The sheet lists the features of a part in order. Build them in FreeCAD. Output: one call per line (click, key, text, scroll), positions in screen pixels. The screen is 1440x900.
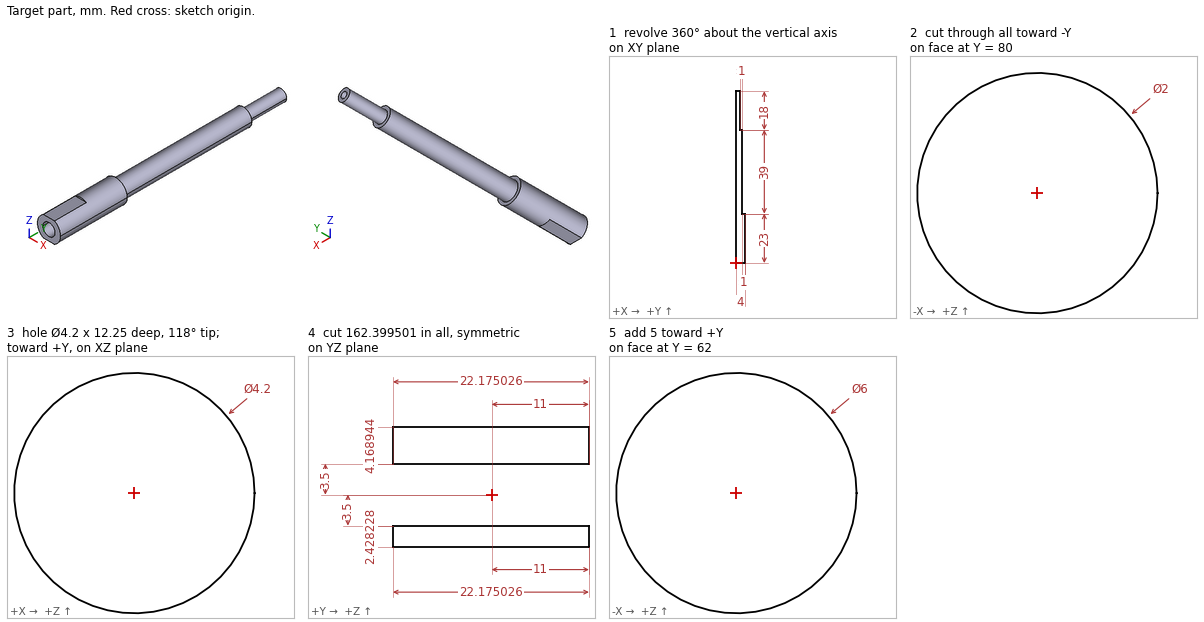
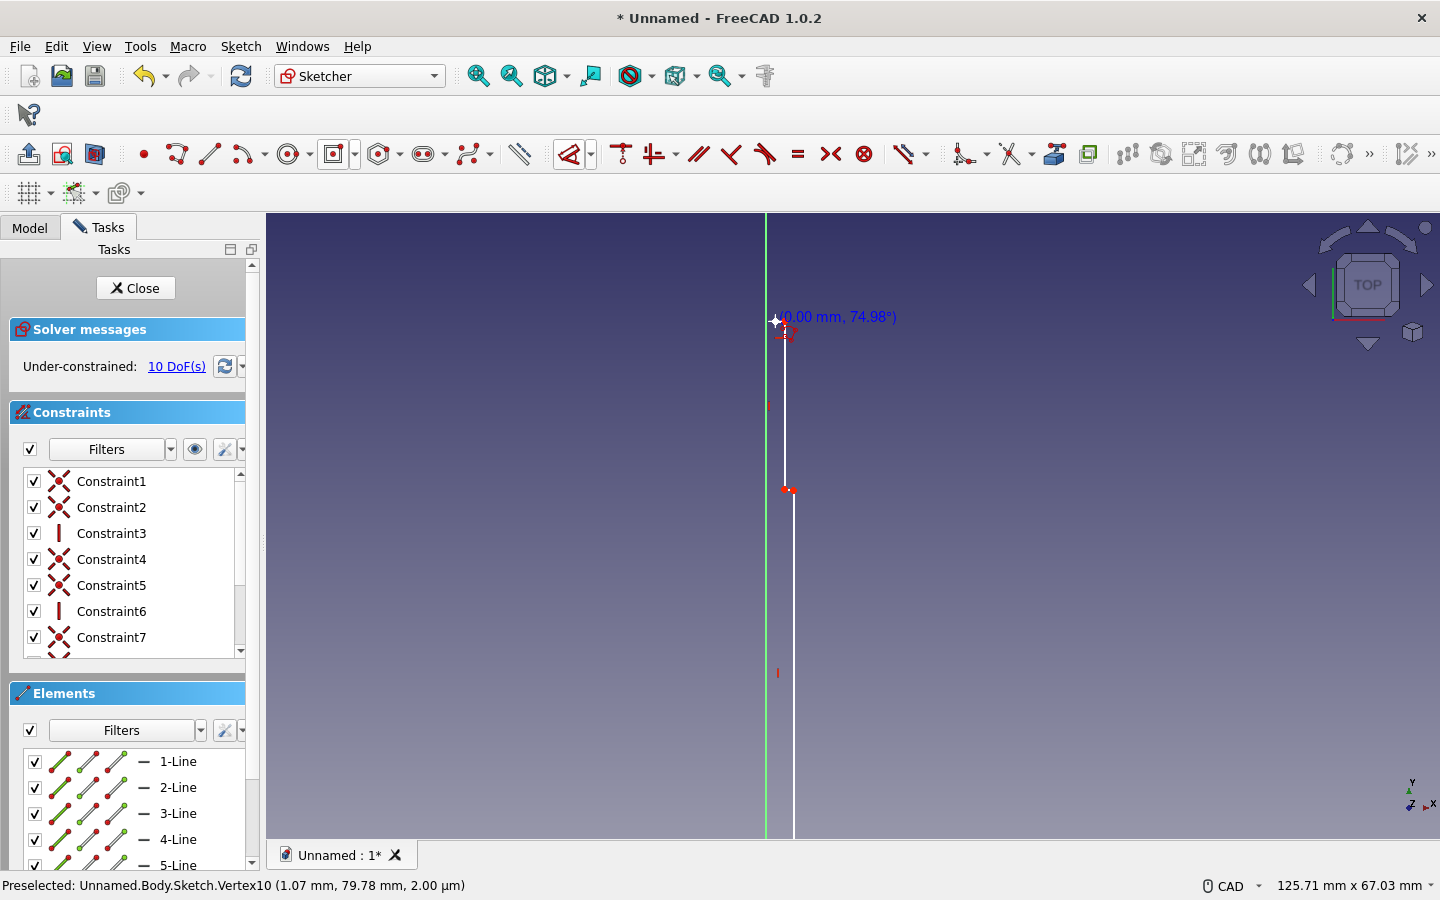
scroll(784, 321, down, 3)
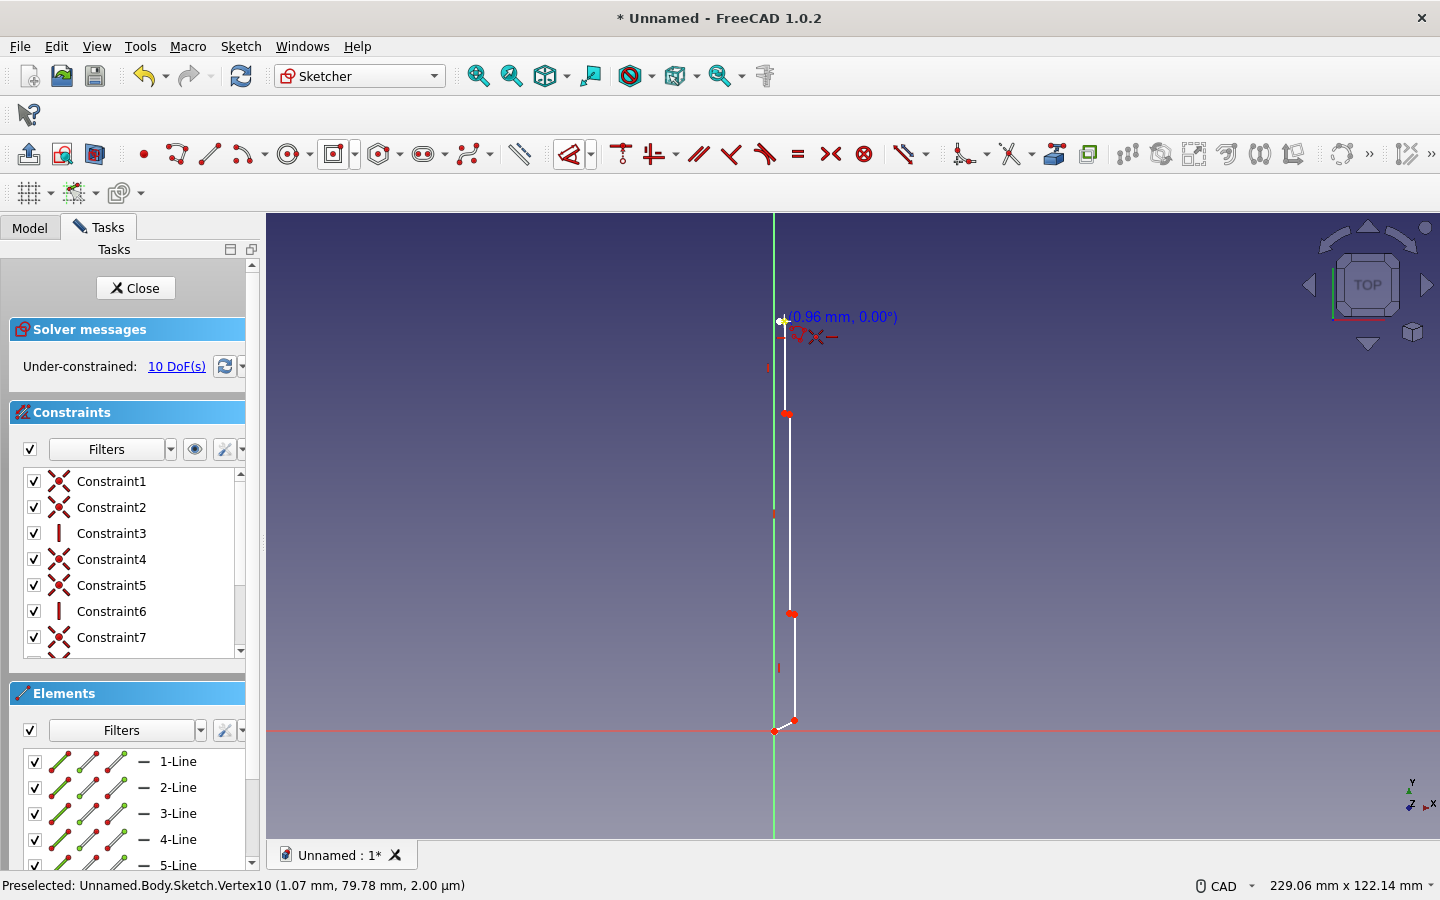
scroll(774, 731, up, 3)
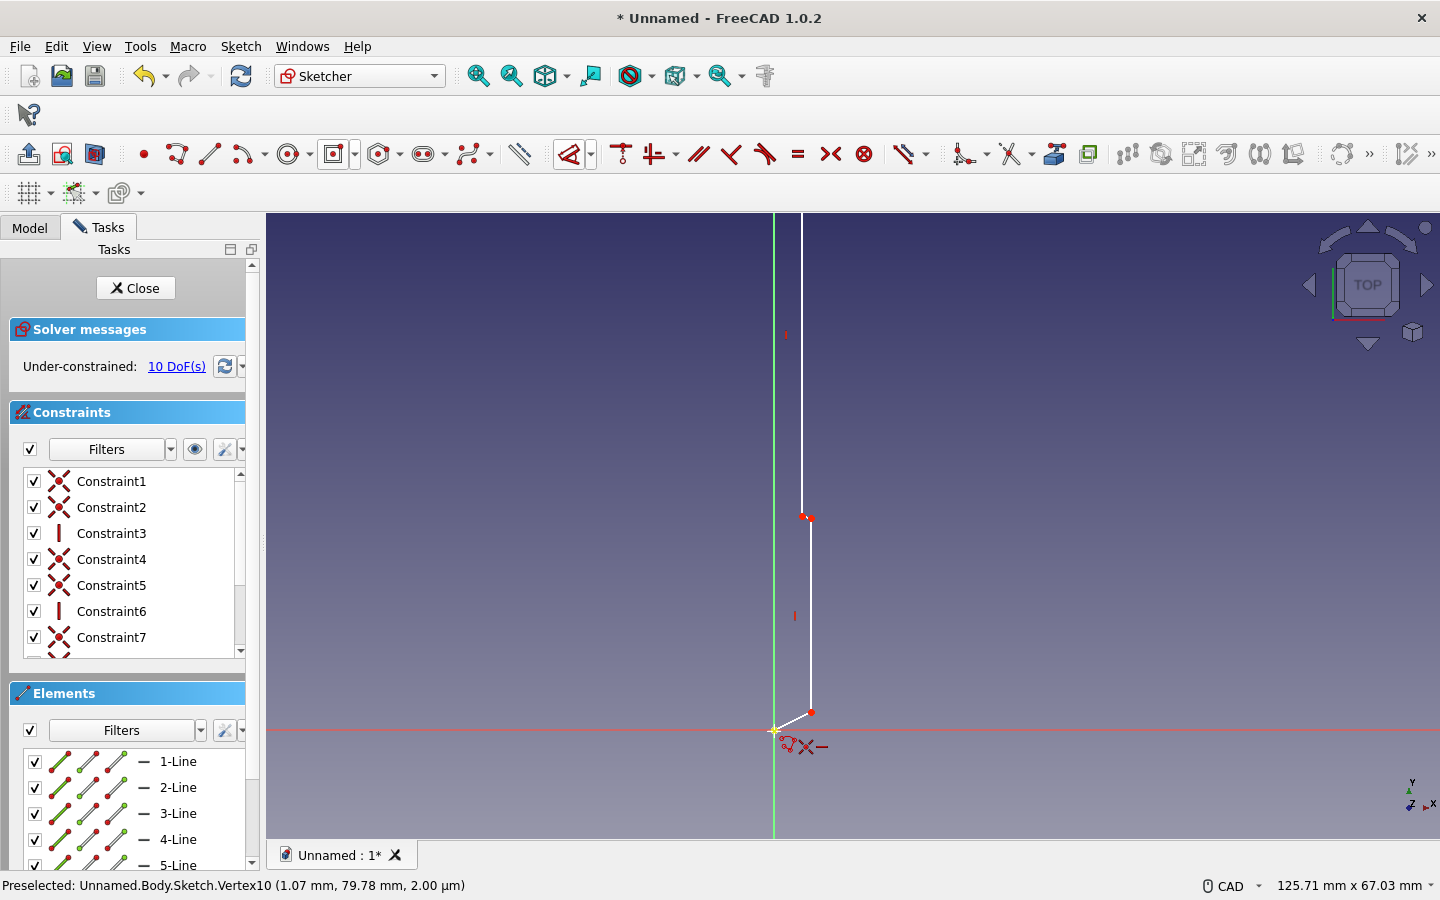
click(774, 730)
key(Escape)
key(Escape)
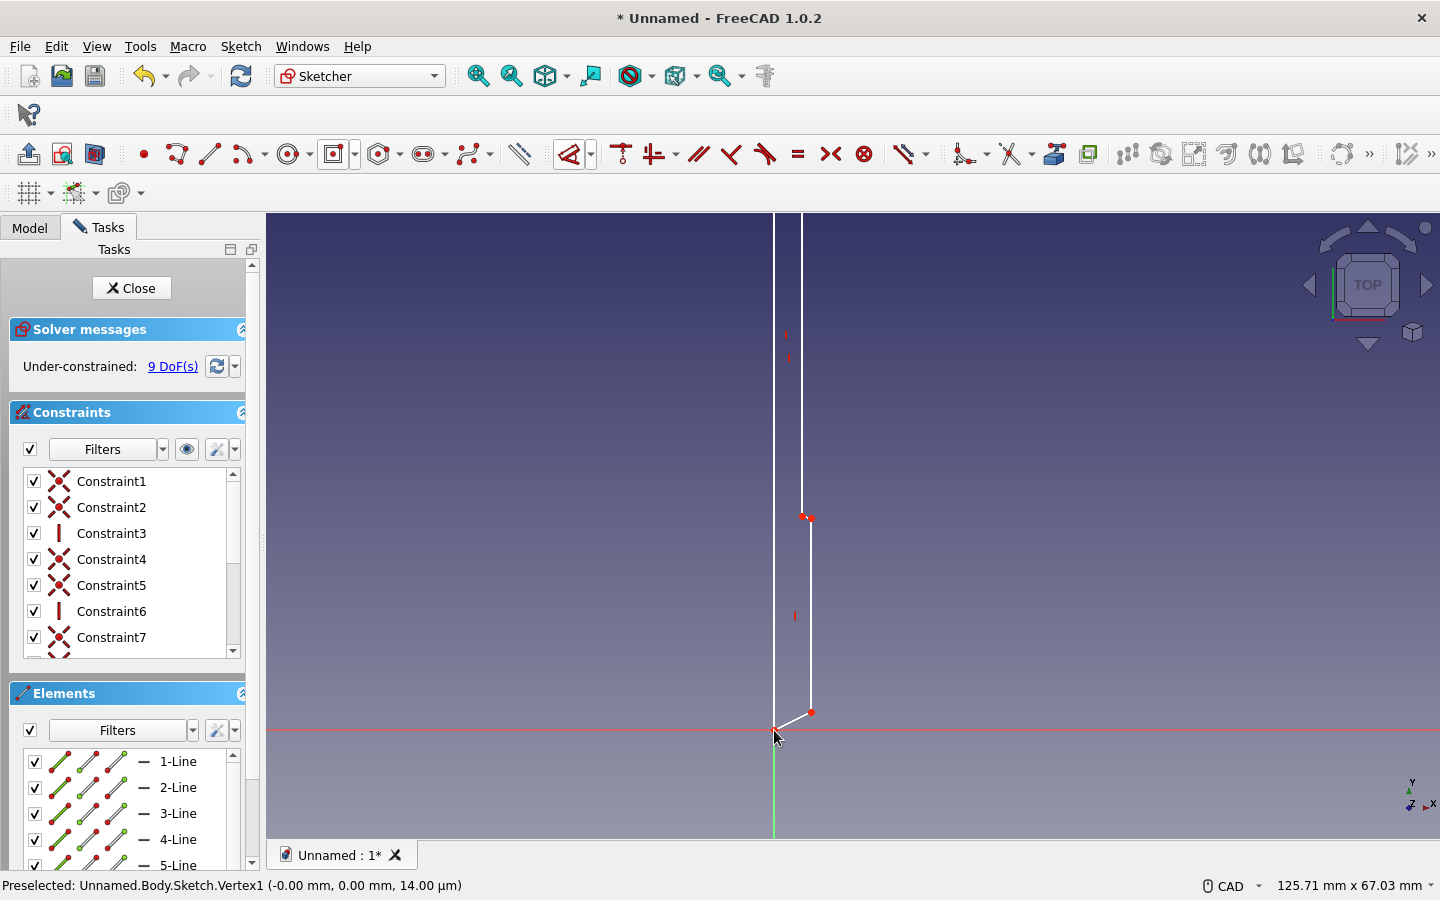
click(800, 718)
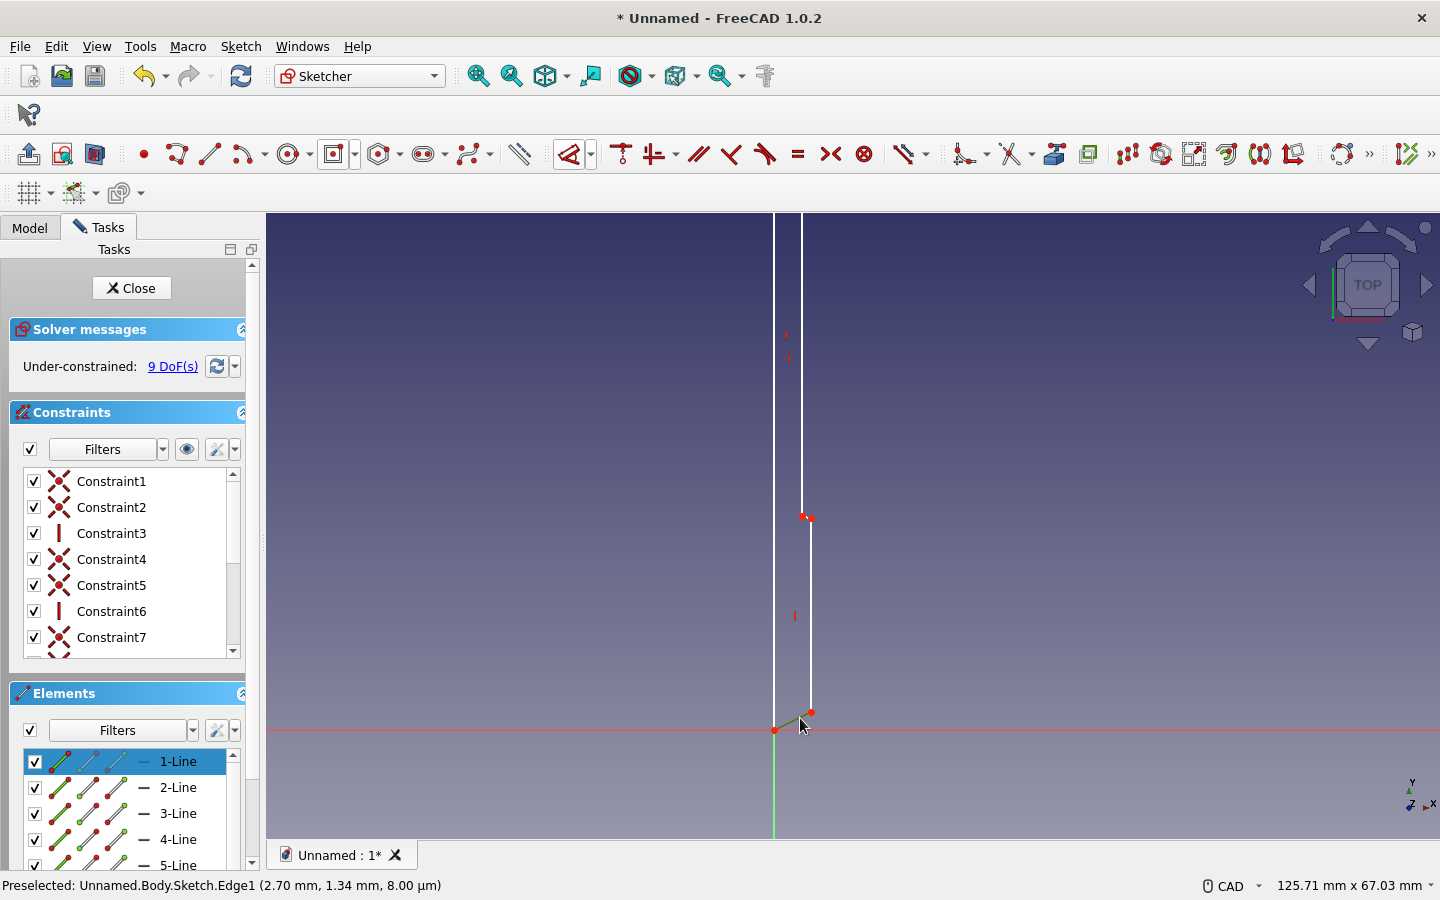
key(h)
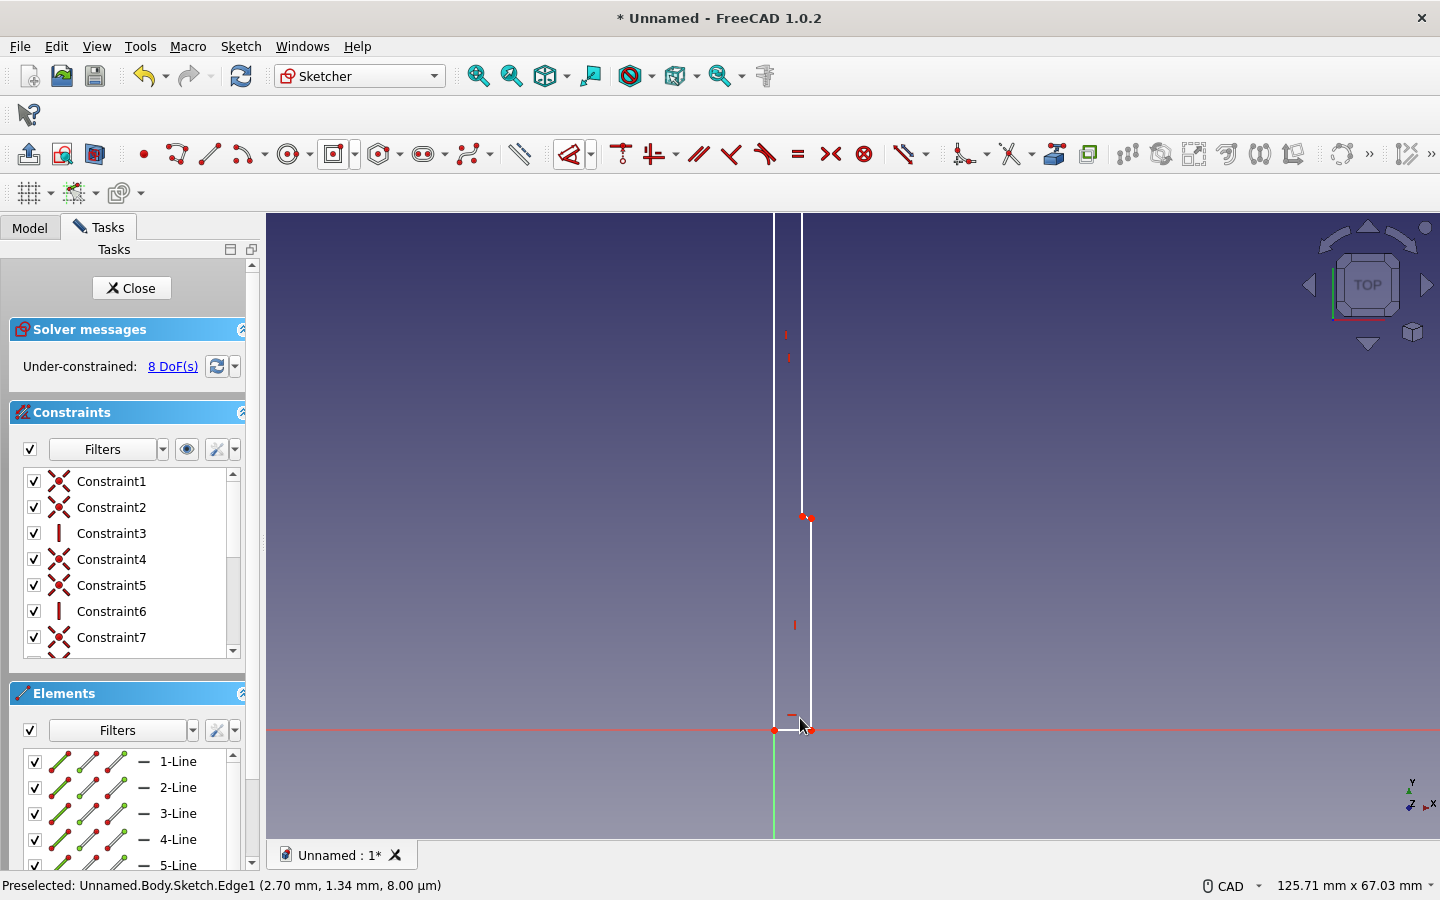
scroll(807, 517, up, 6)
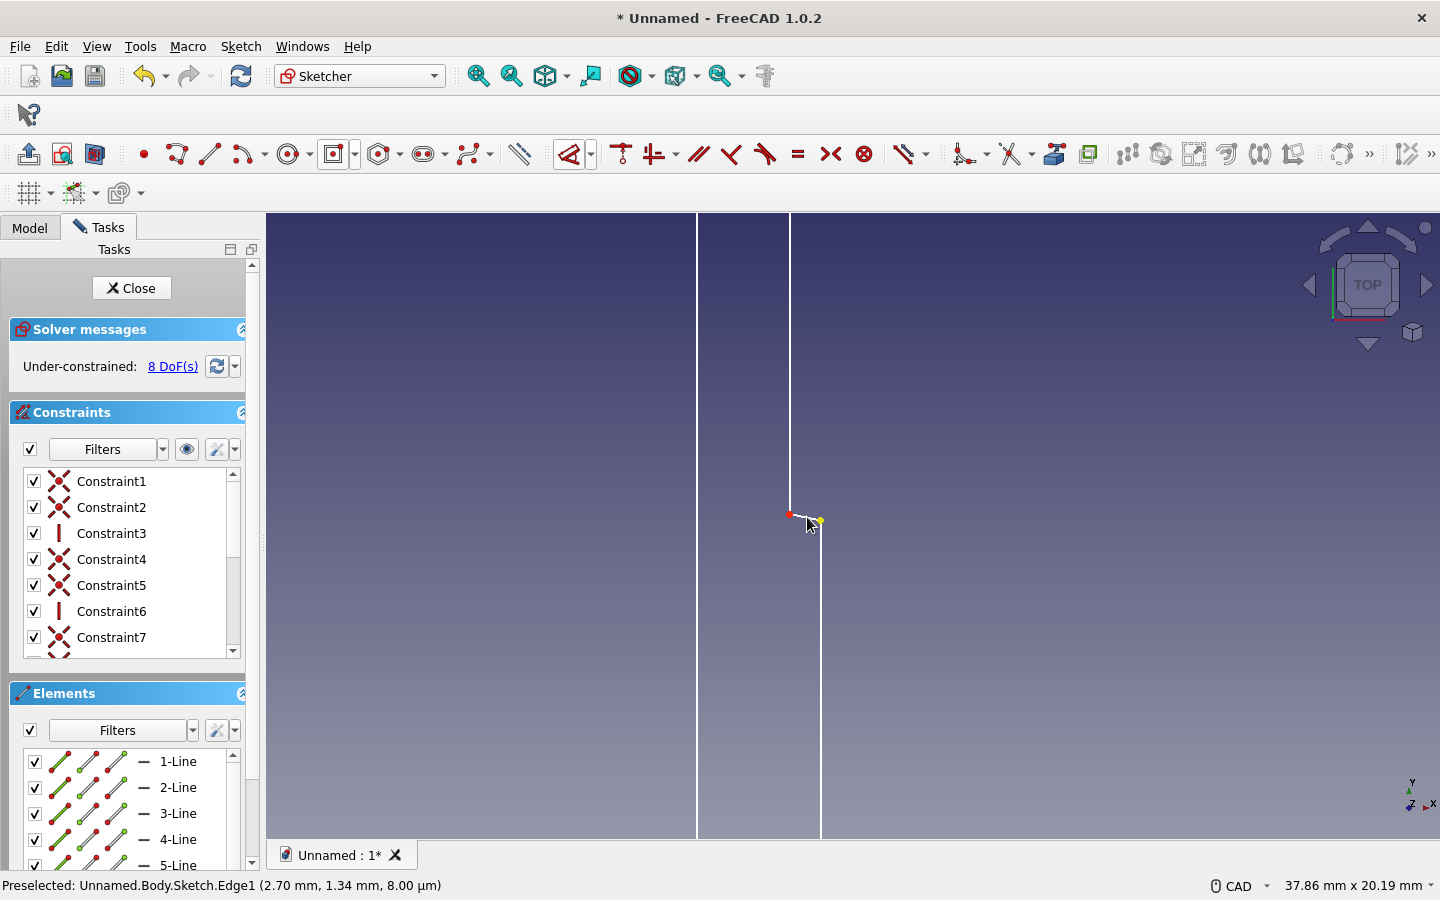
click(805, 517)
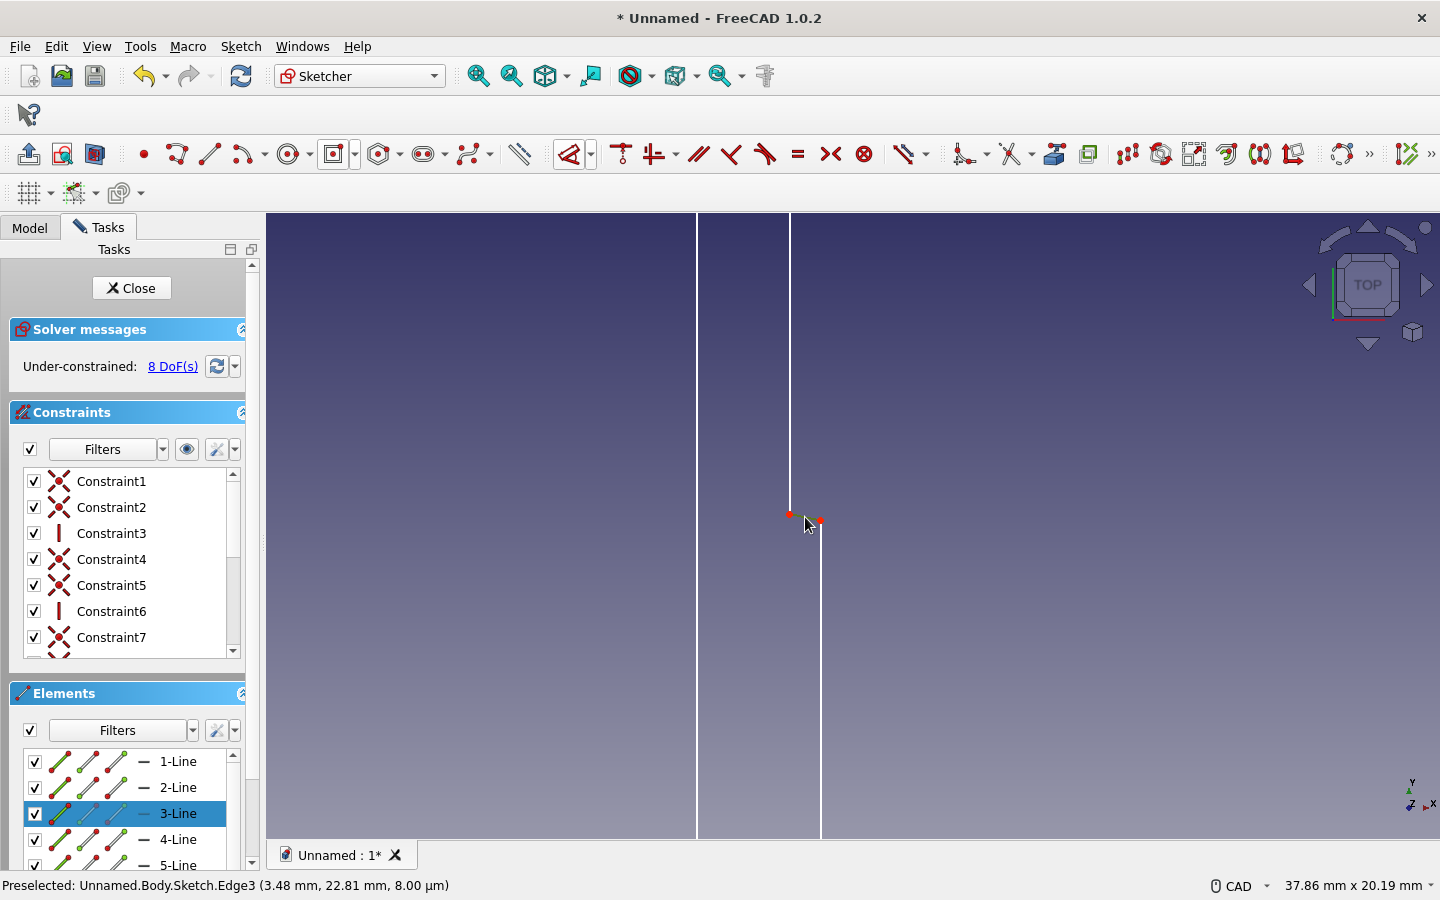
key(h)